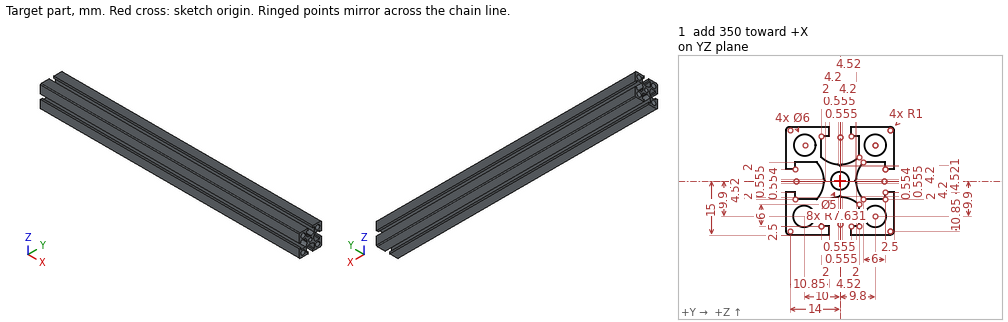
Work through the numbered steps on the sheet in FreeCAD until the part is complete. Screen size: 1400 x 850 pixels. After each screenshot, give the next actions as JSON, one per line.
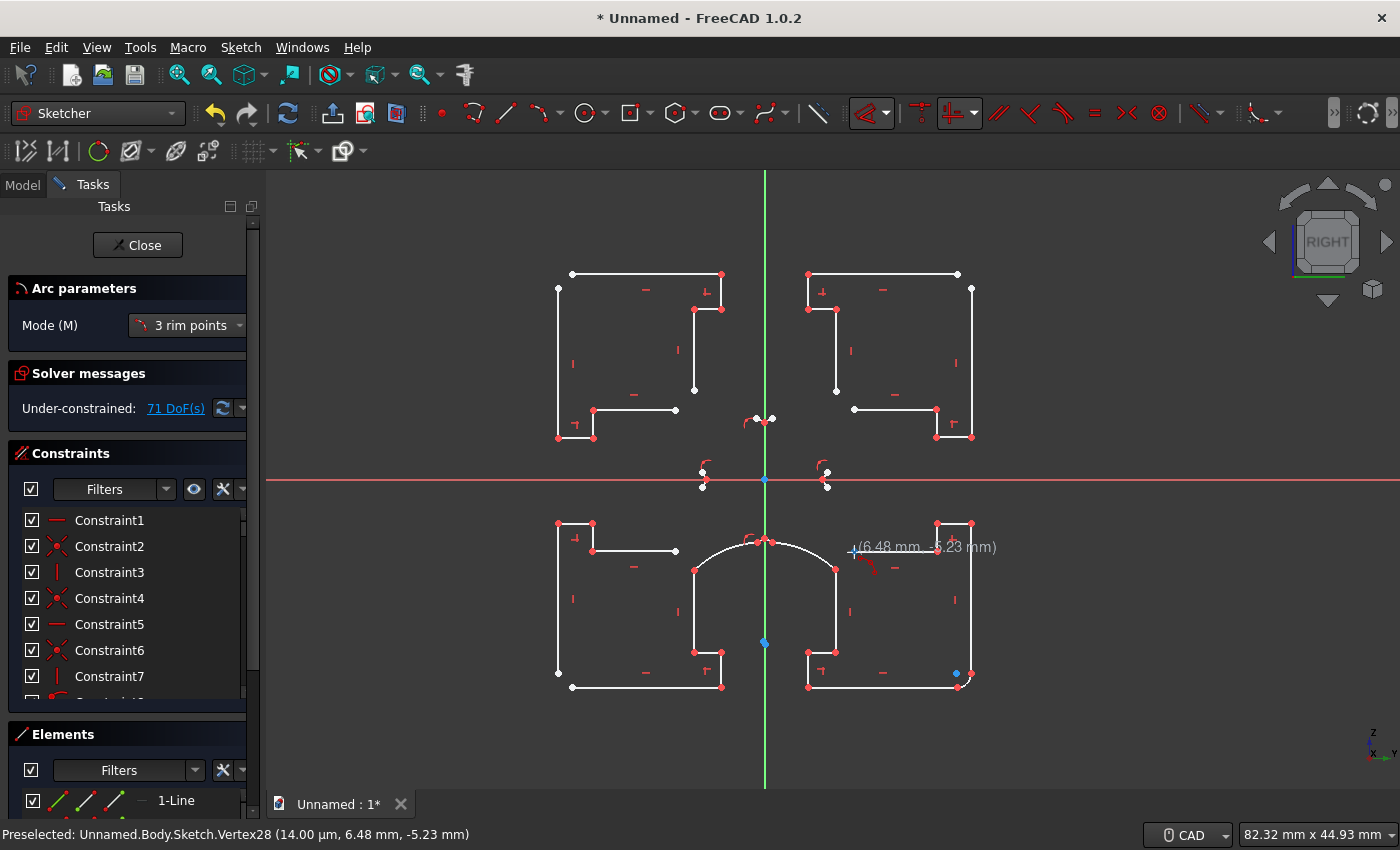
{"action": "scroll", "coordinate": [827, 488], "scroll_direction": "up", "scroll_amount": 7}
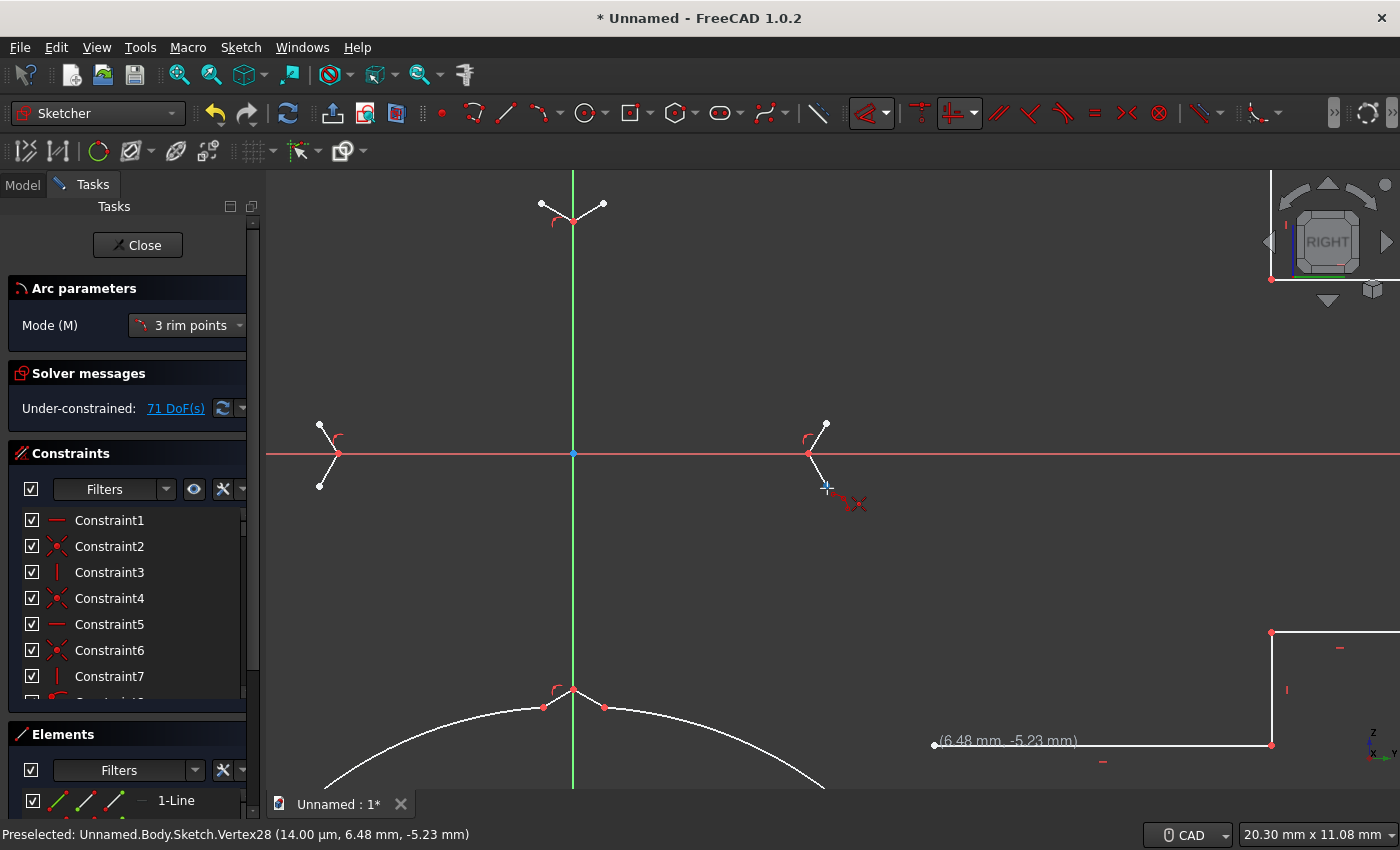
{"action": "left_click", "coordinate": [827, 486]}
{"action": "left_click", "coordinate": [859, 622]}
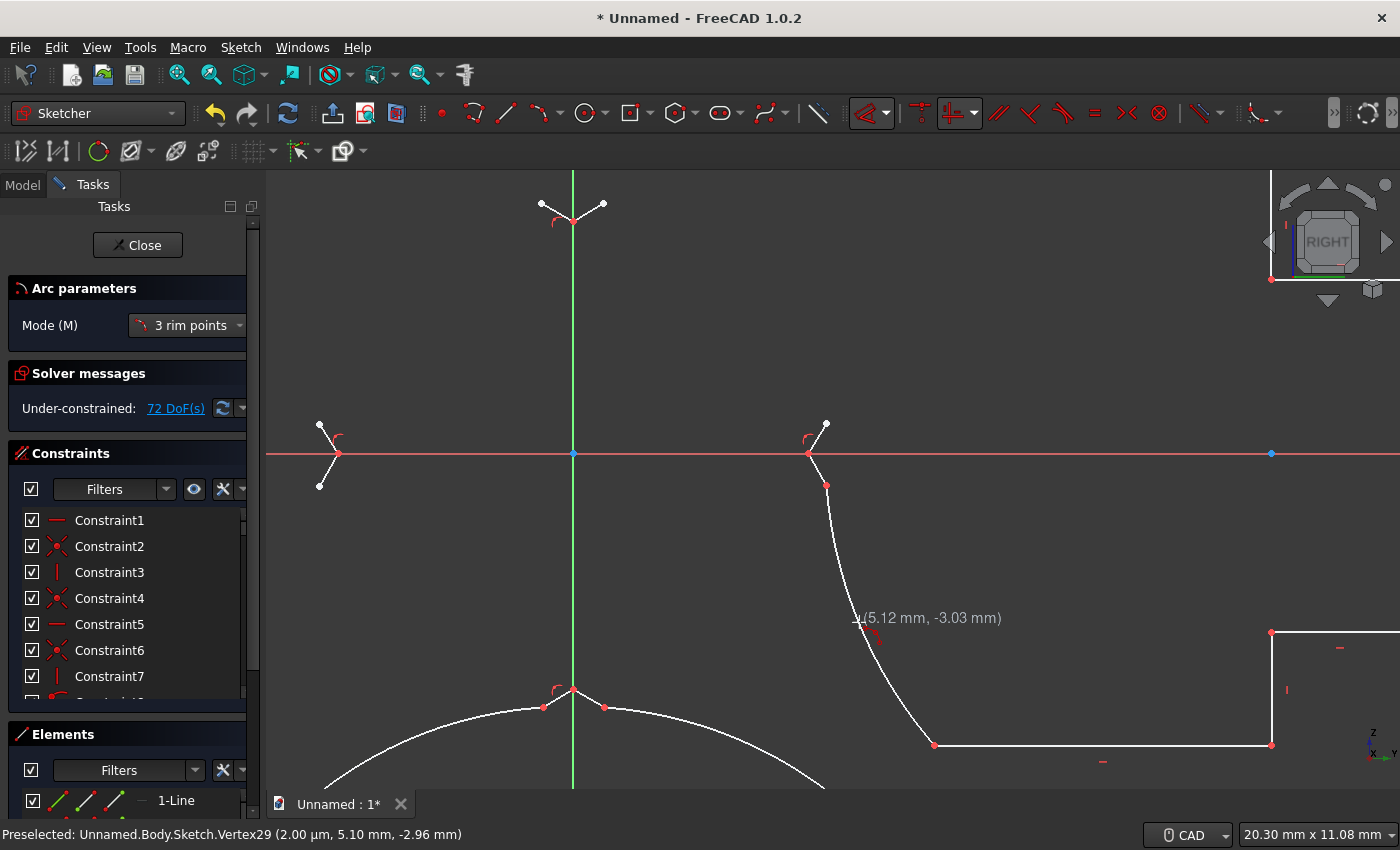
{"action": "left_click", "coordinate": [827, 424]}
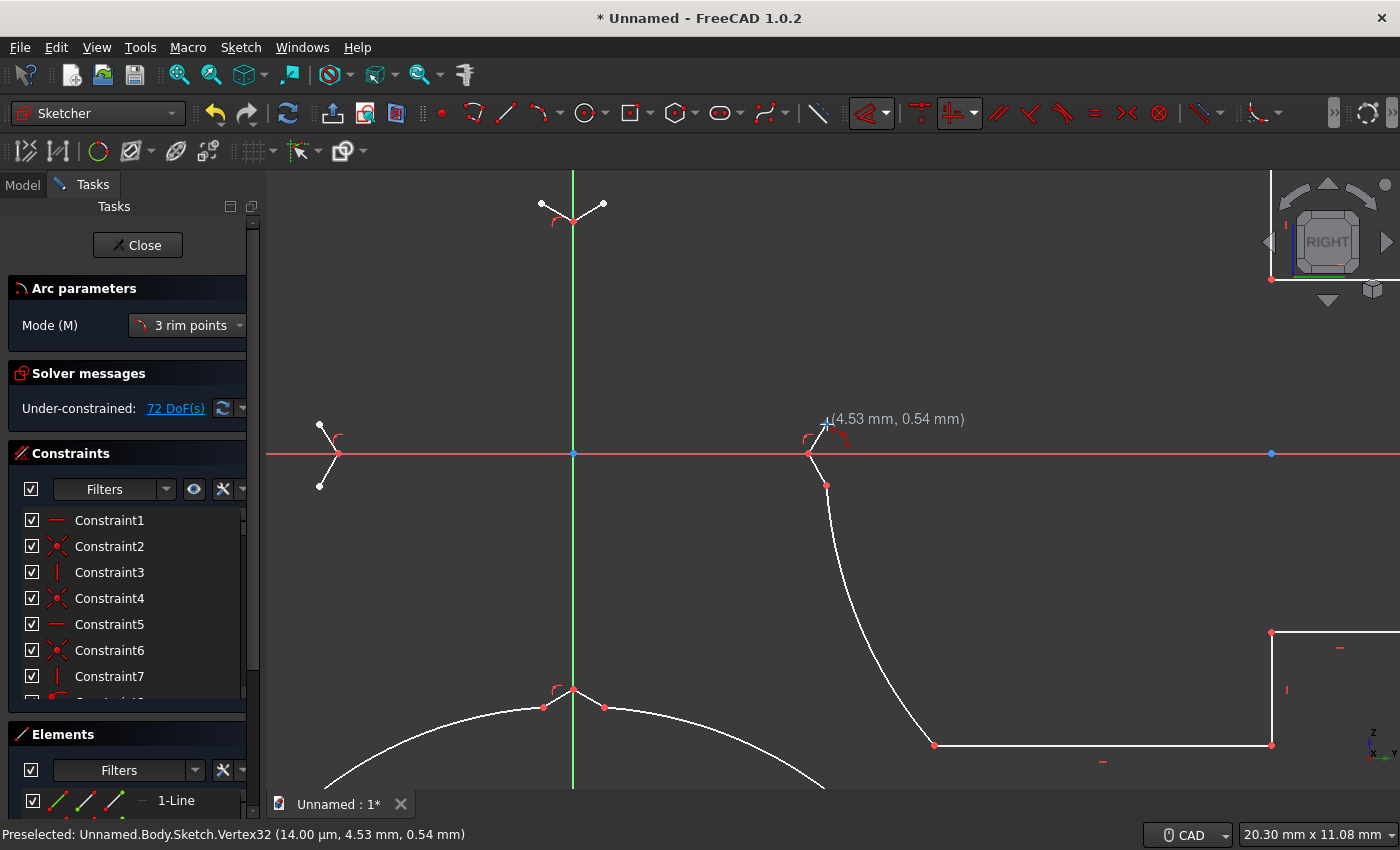
{"action": "scroll", "coordinate": [827, 488], "scroll_direction": "down", "scroll_amount": 7}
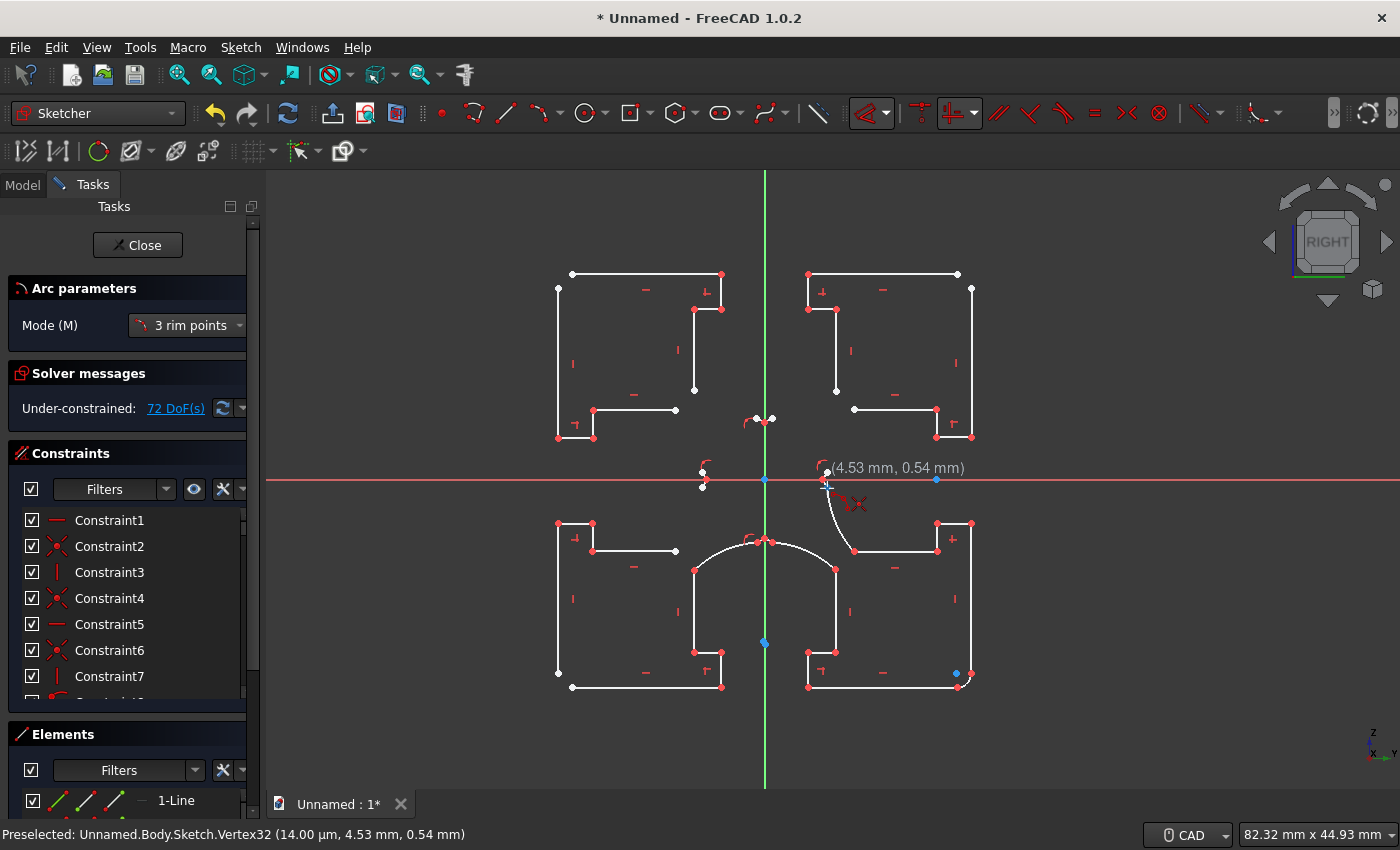
{"action": "left_click", "coordinate": [854, 410]}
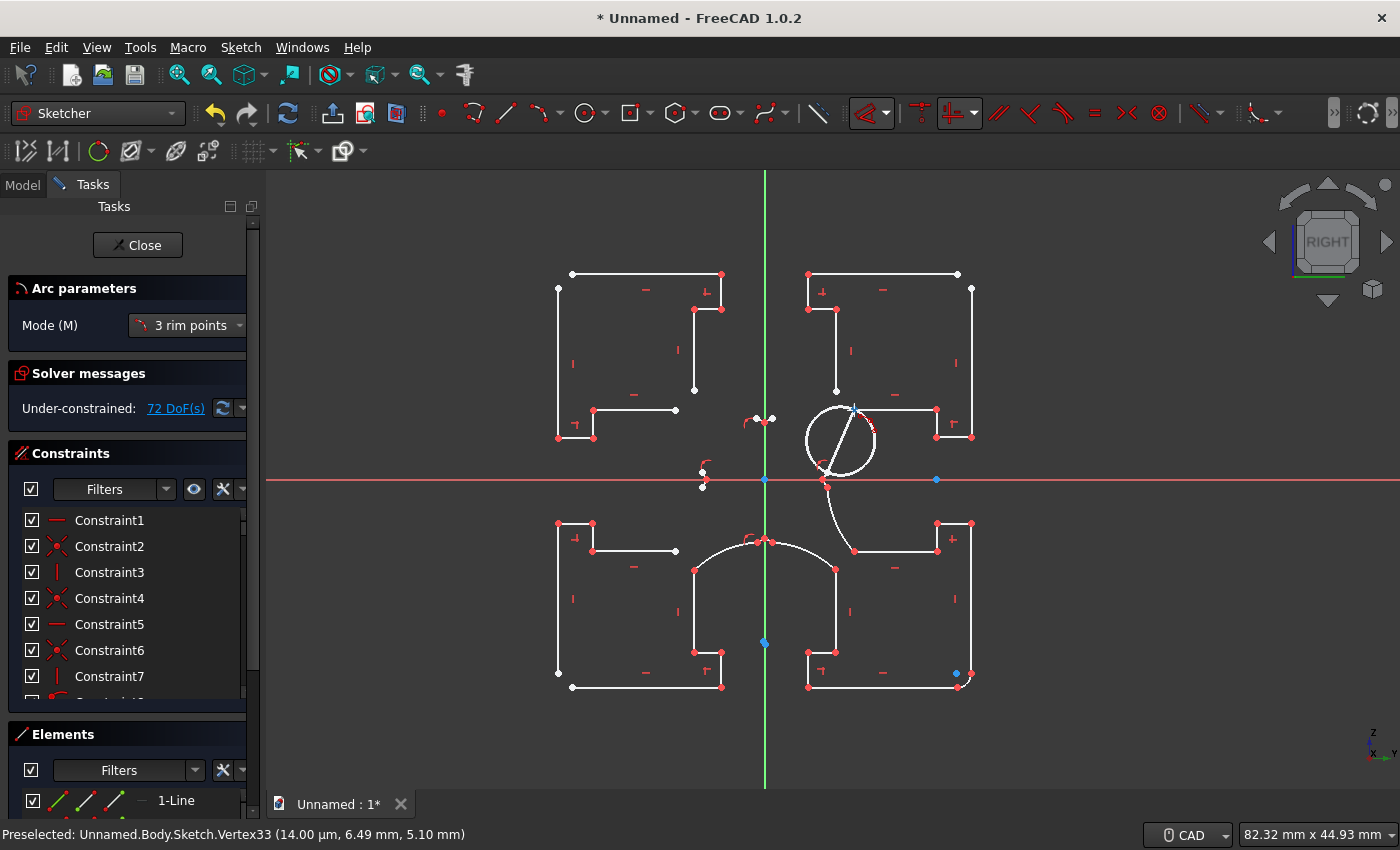
{"action": "scroll", "coordinate": [835, 438], "scroll_direction": "up", "scroll_amount": 6}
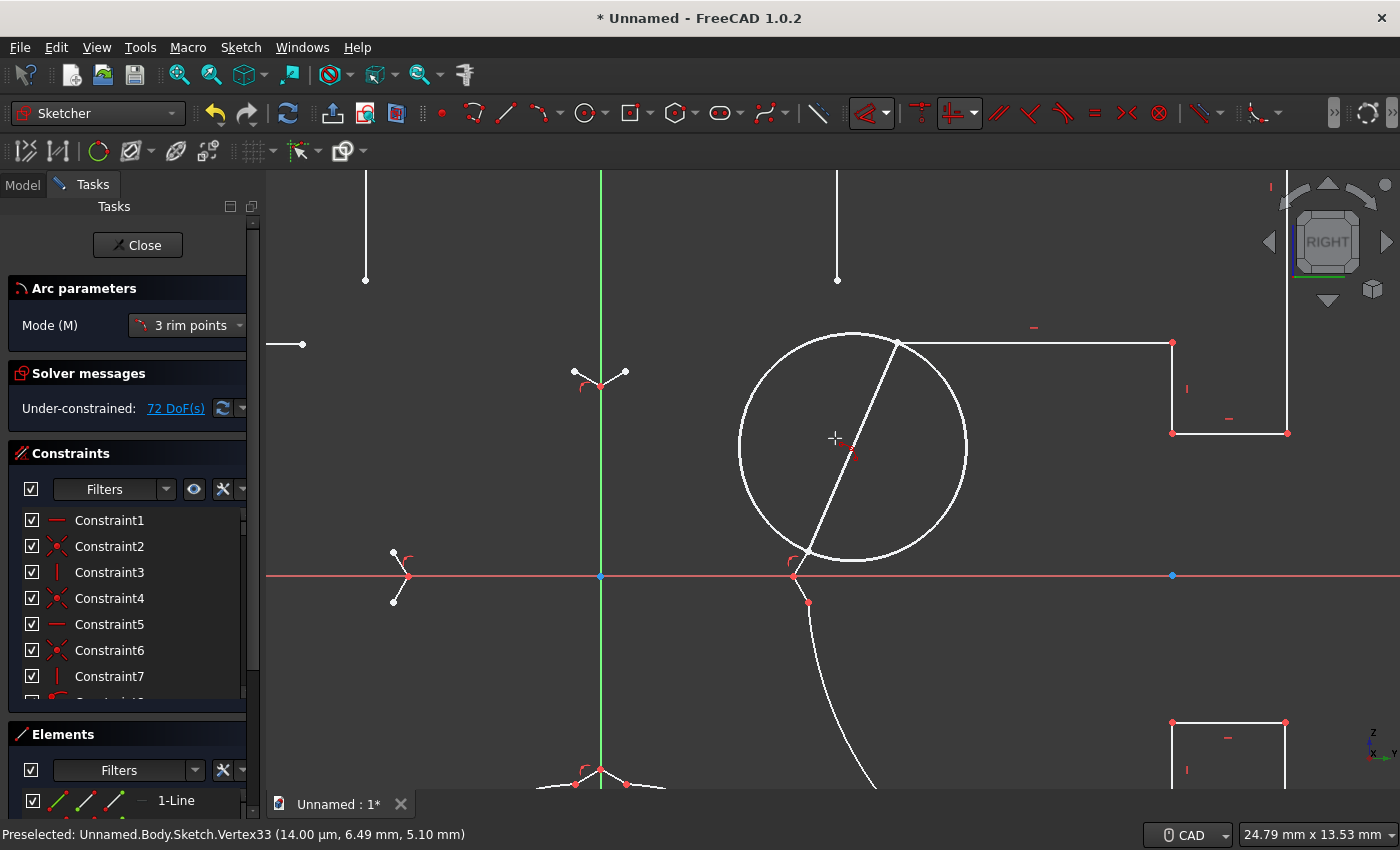
{"action": "left_click", "coordinate": [835, 438]}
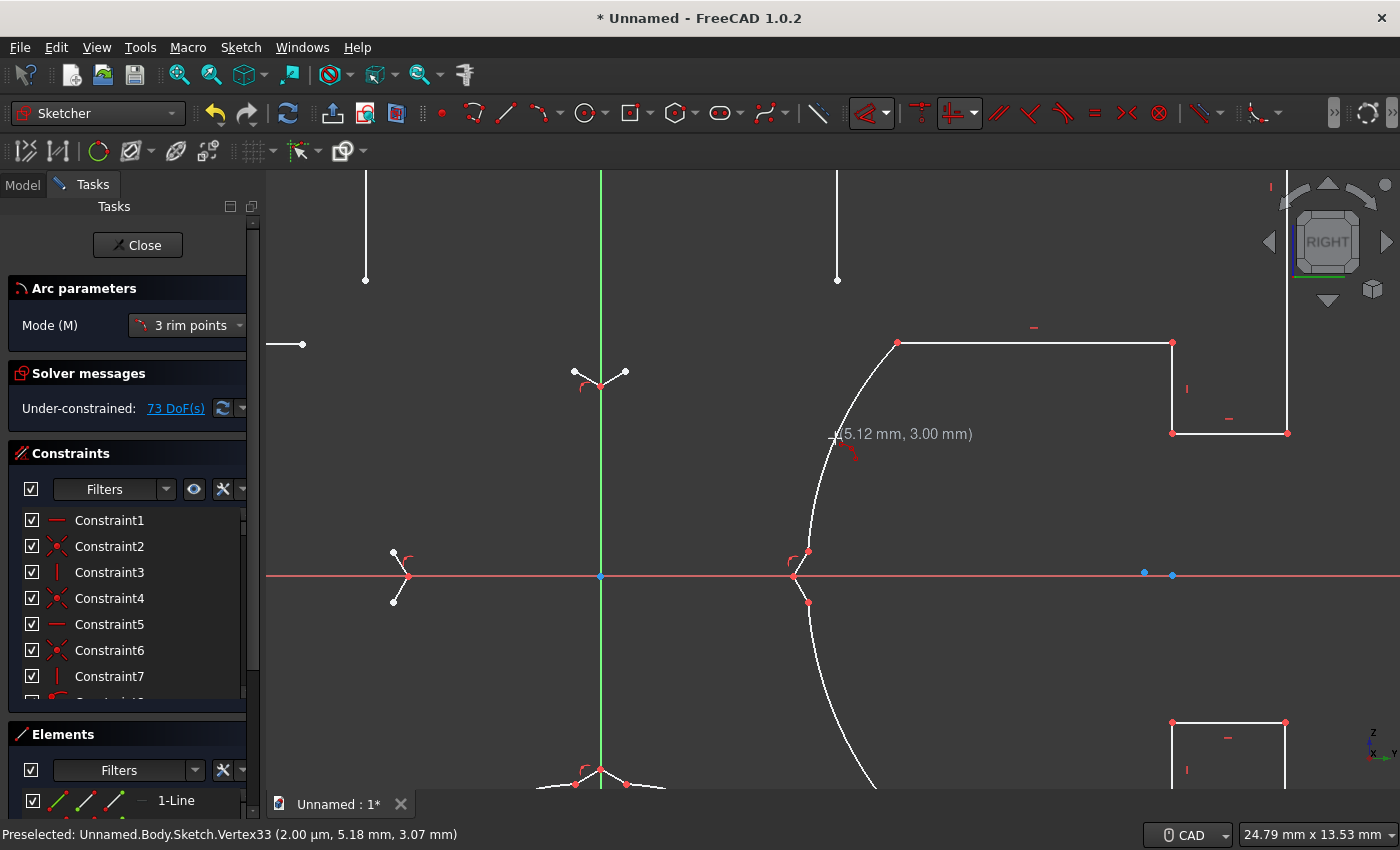
{"action": "scroll", "coordinate": [835, 438], "scroll_direction": "down", "scroll_amount": 6}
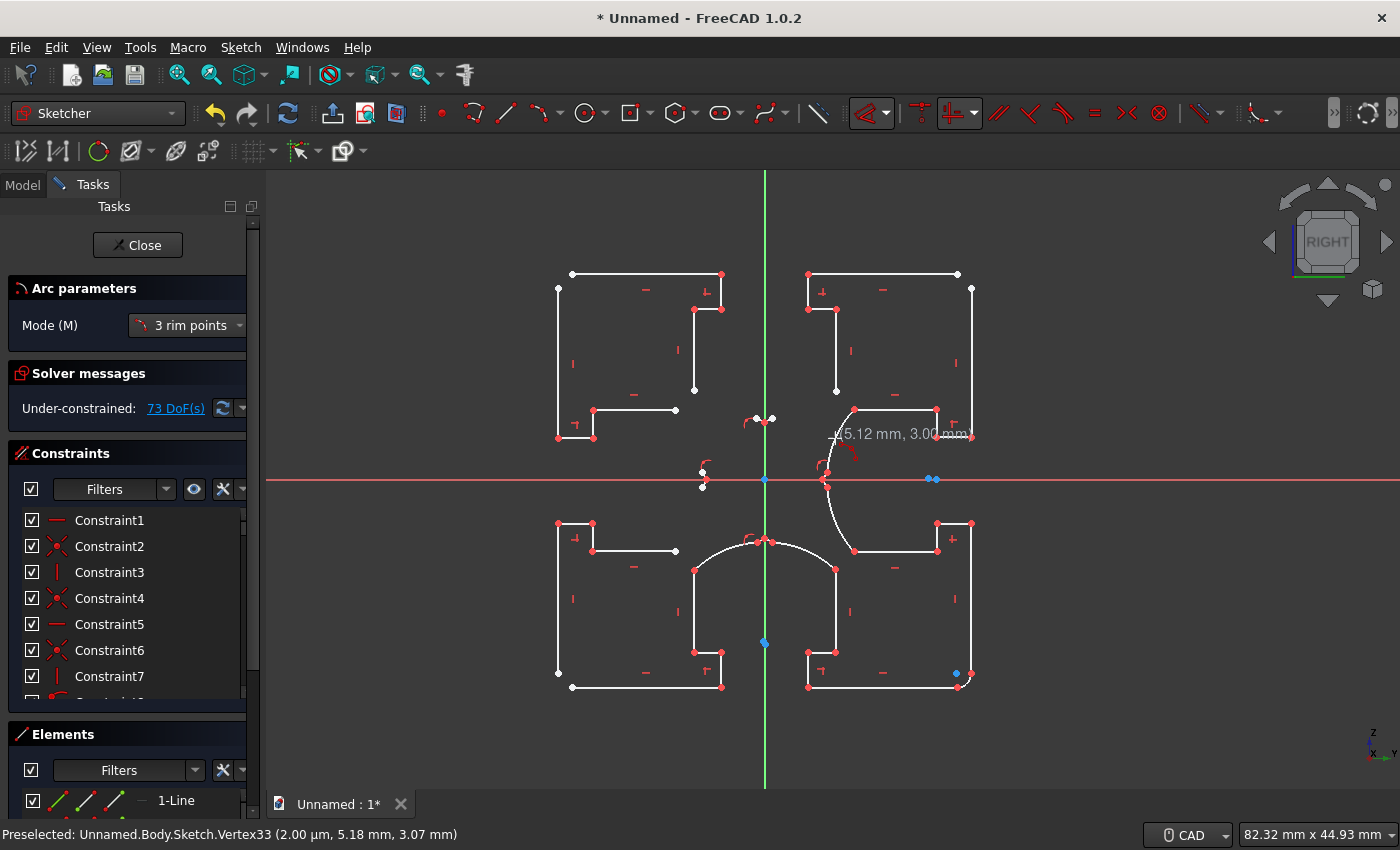
{"action": "left_click", "coordinate": [972, 288]}
{"action": "left_click", "coordinate": [958, 274]}